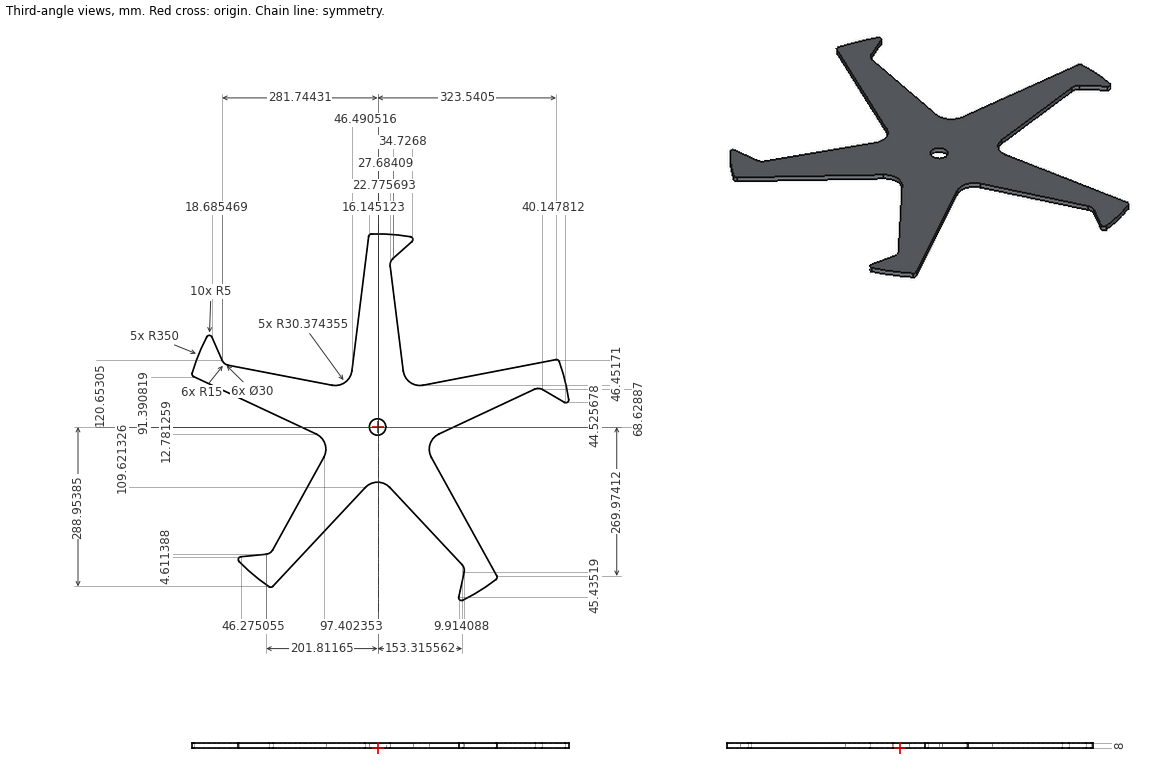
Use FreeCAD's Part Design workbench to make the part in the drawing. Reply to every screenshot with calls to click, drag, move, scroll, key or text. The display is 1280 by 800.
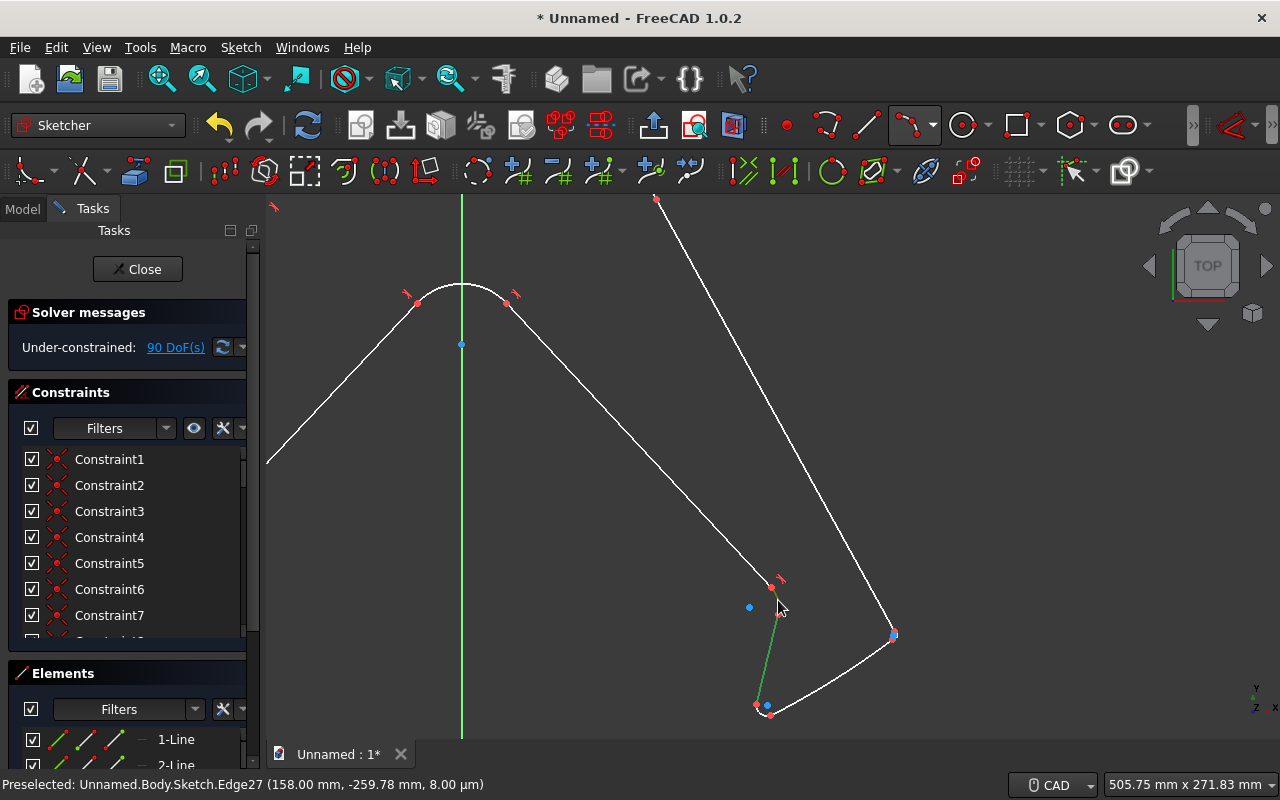
key(t)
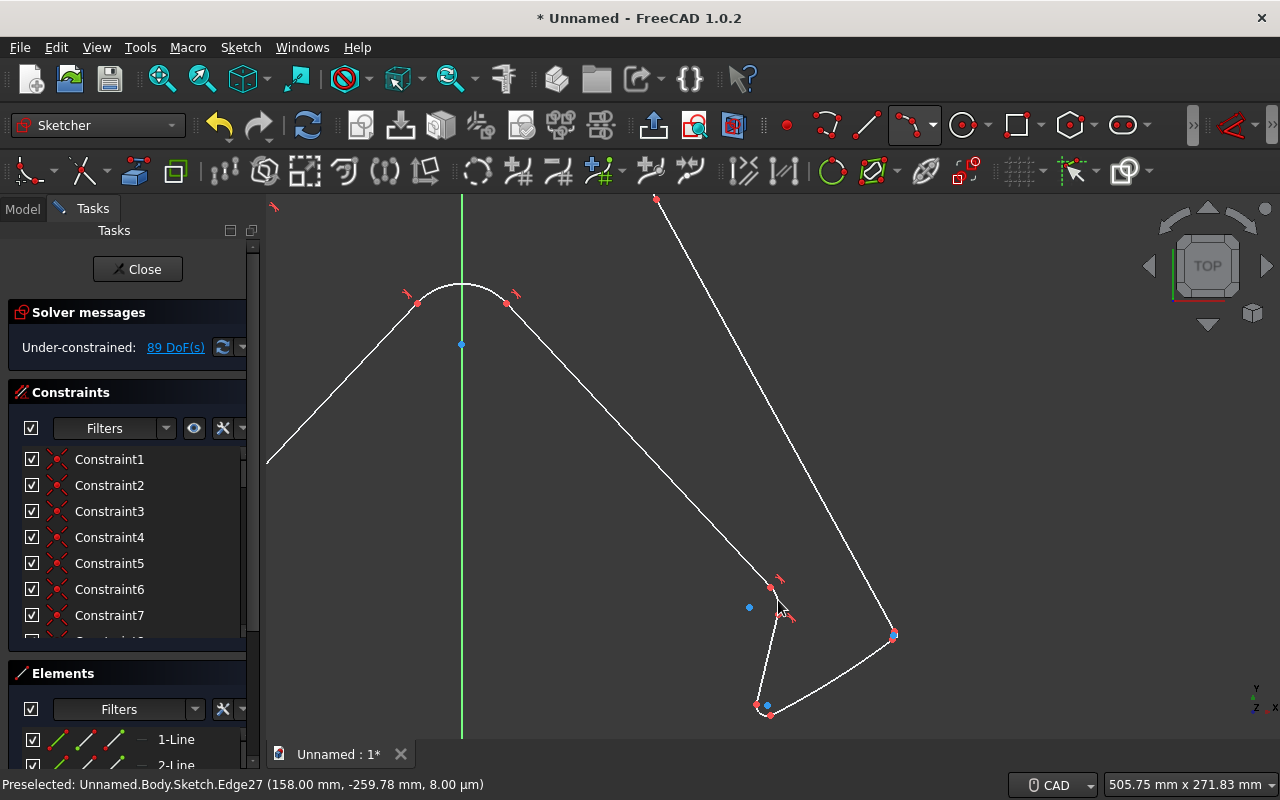
click(772, 641)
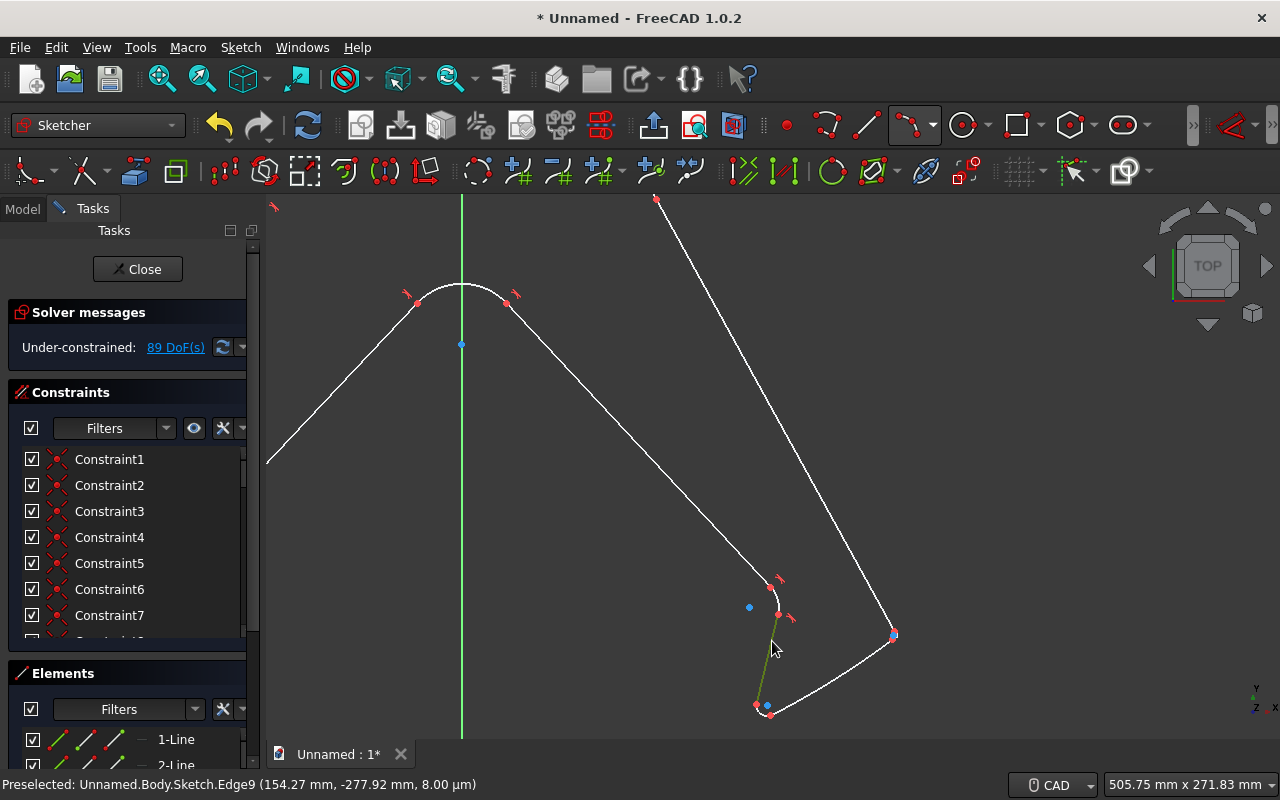
scroll(780, 603, down, 7)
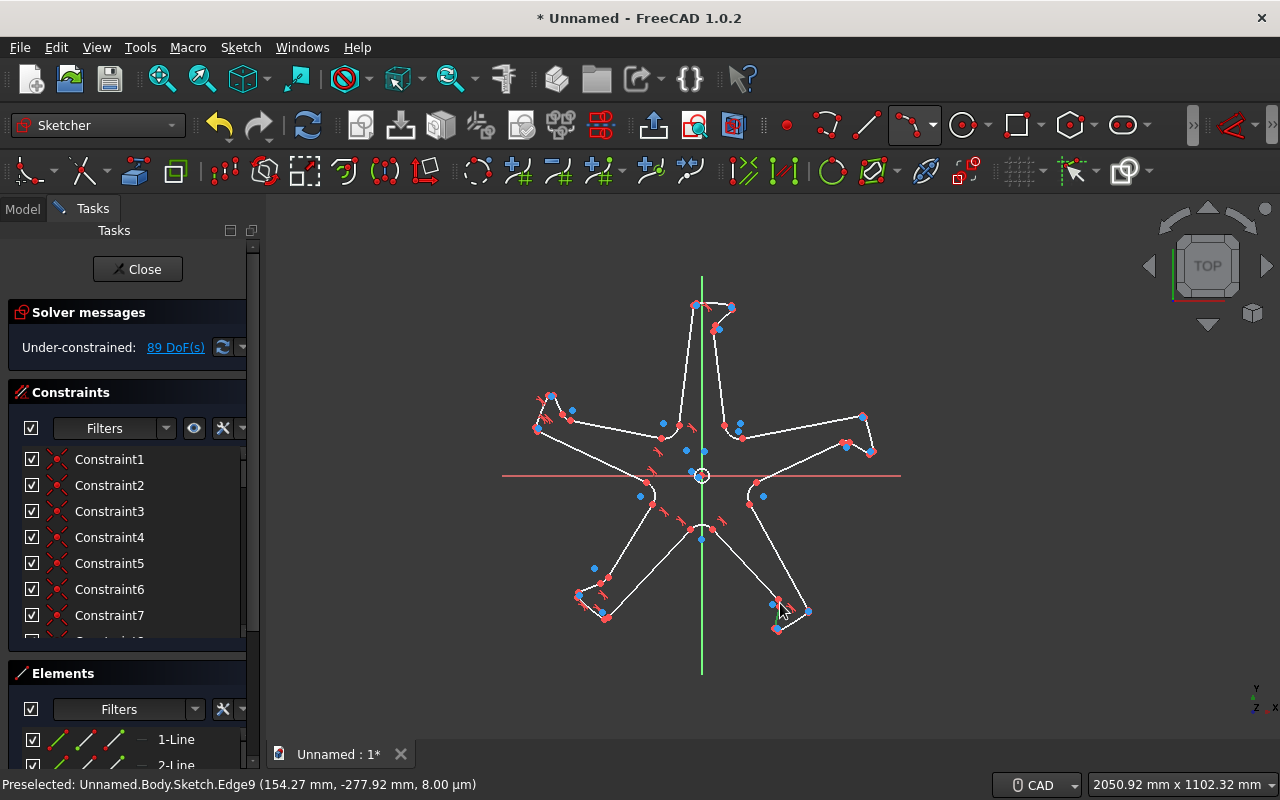
scroll(776, 631, up, 9)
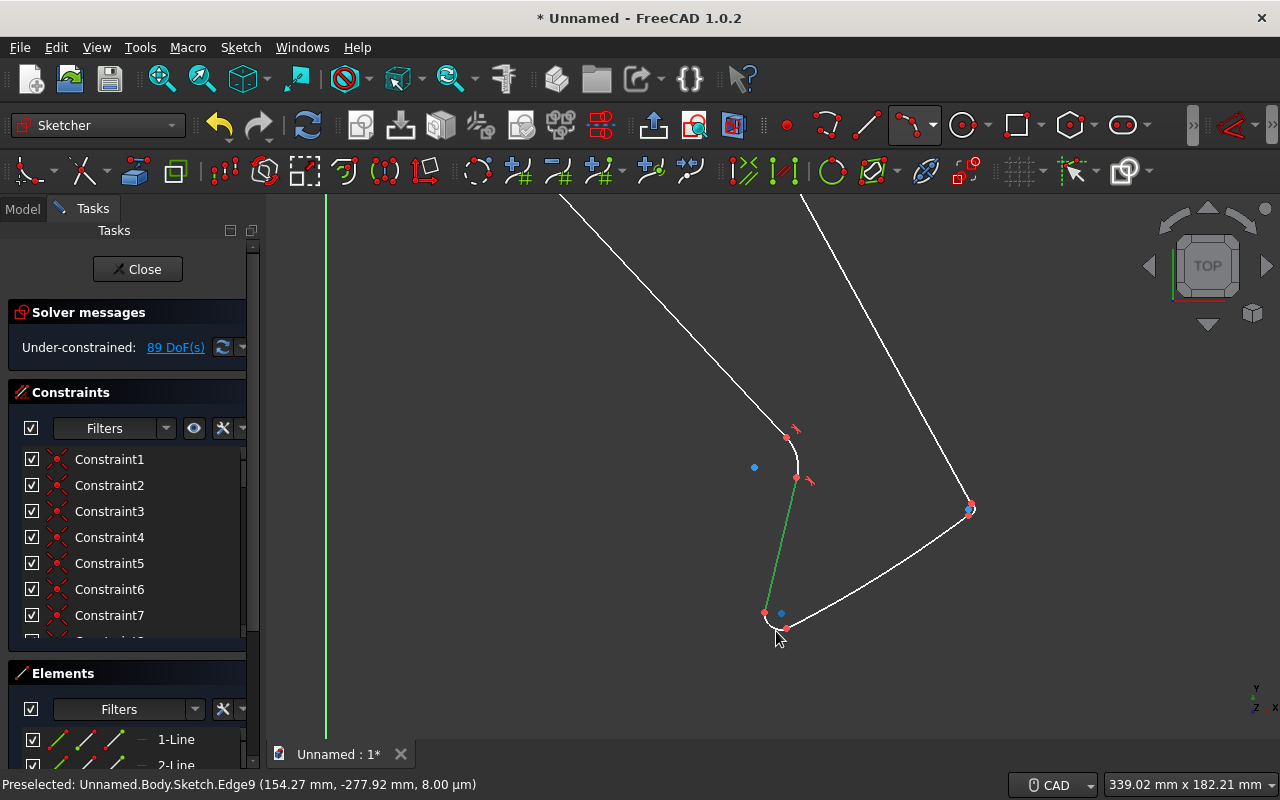
click(771, 627)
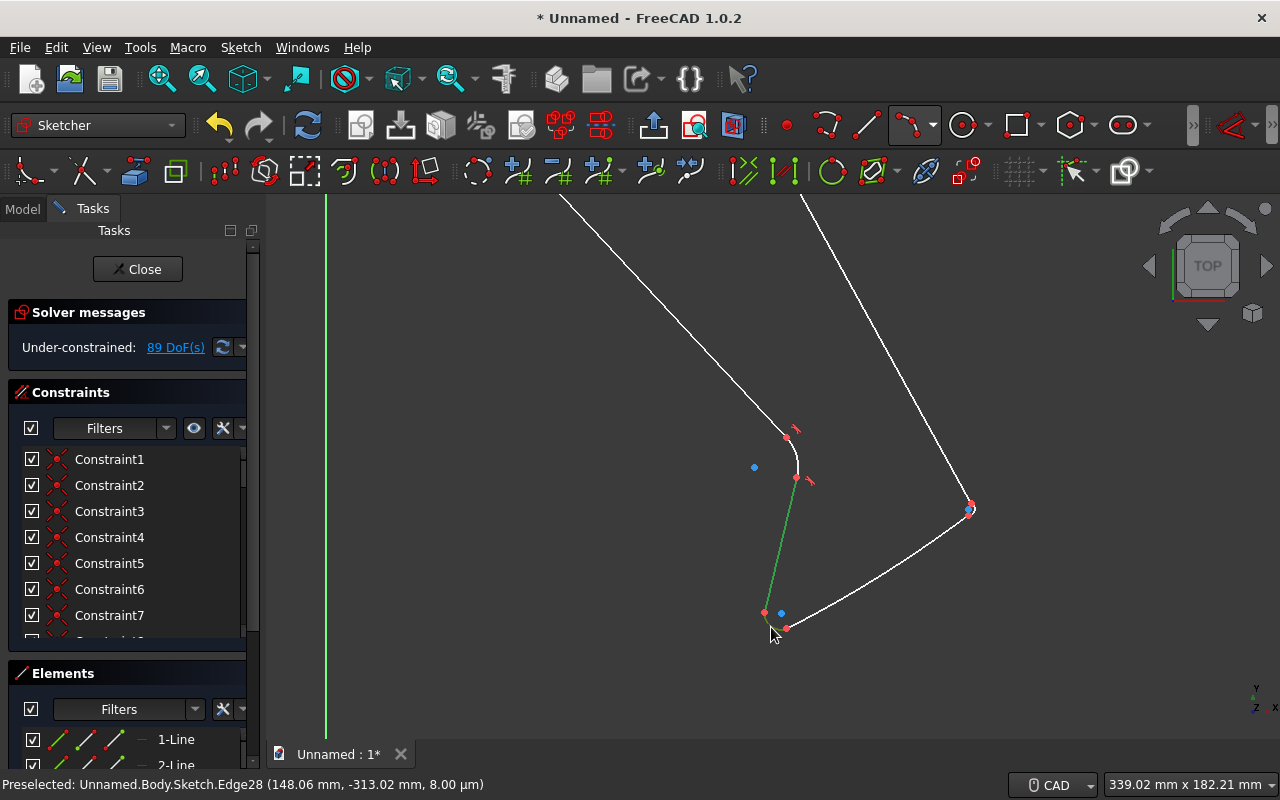
key(t)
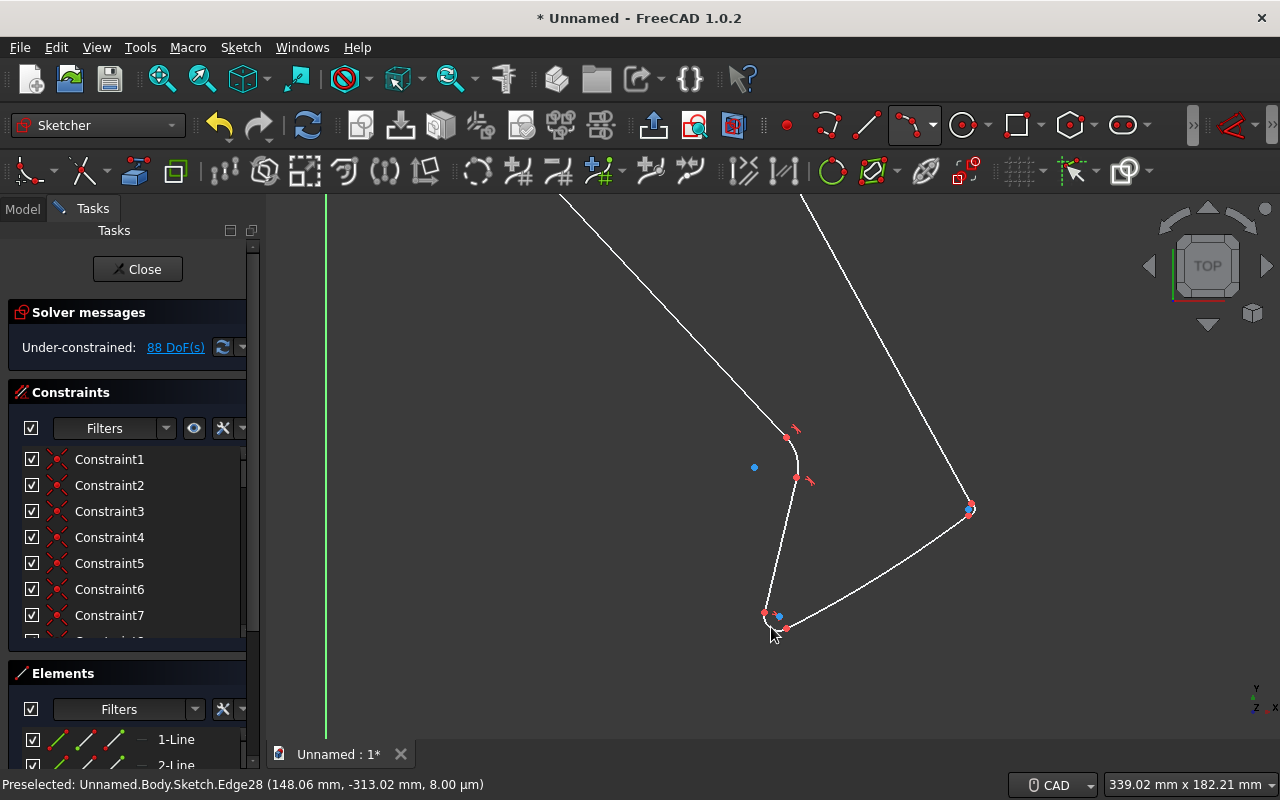
scroll(776, 631, down, 9)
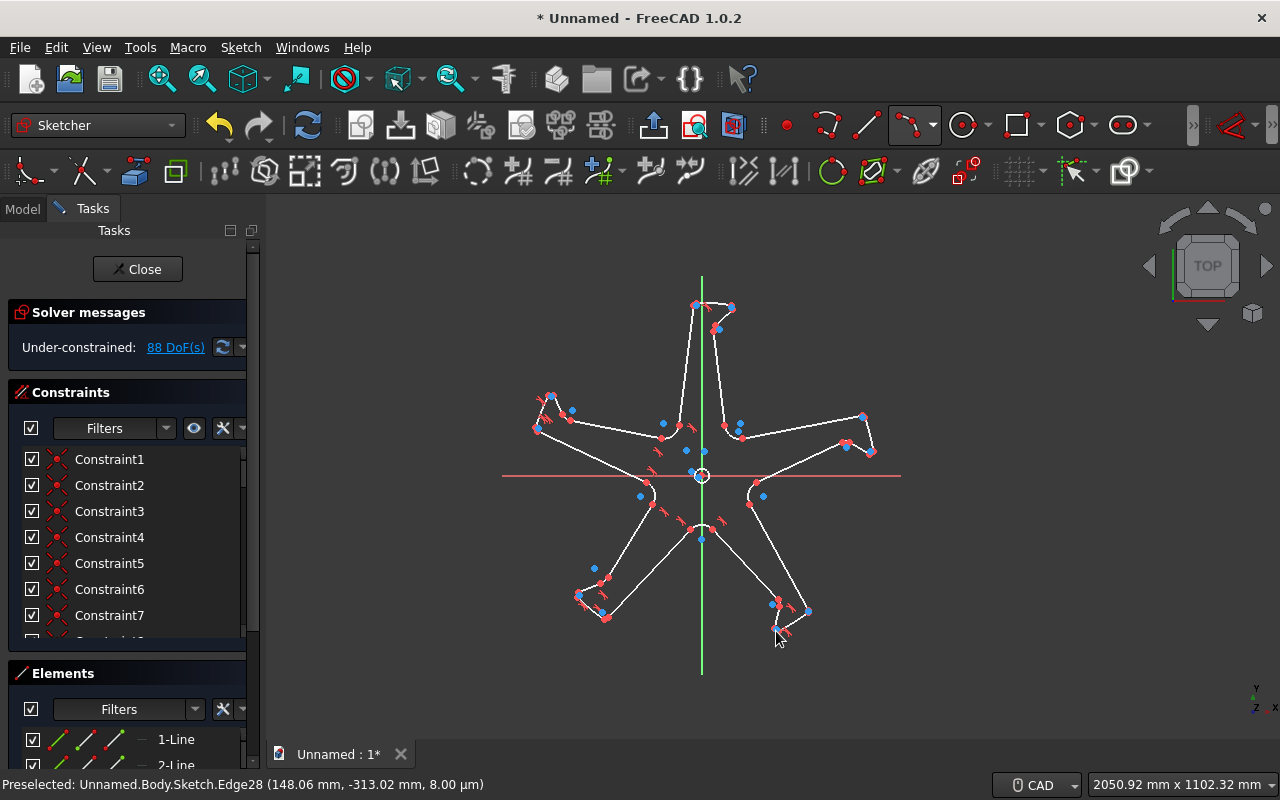
click(791, 579)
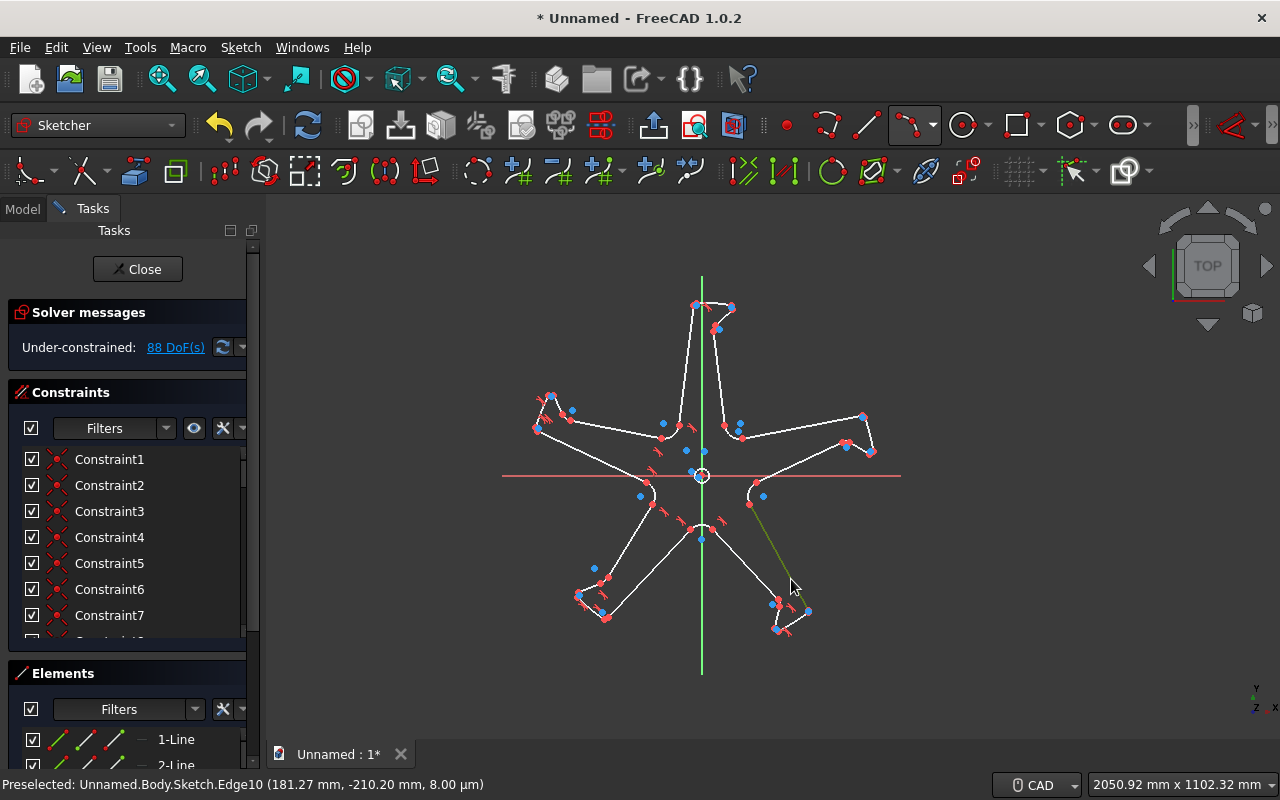
scroll(809, 612, up, 14)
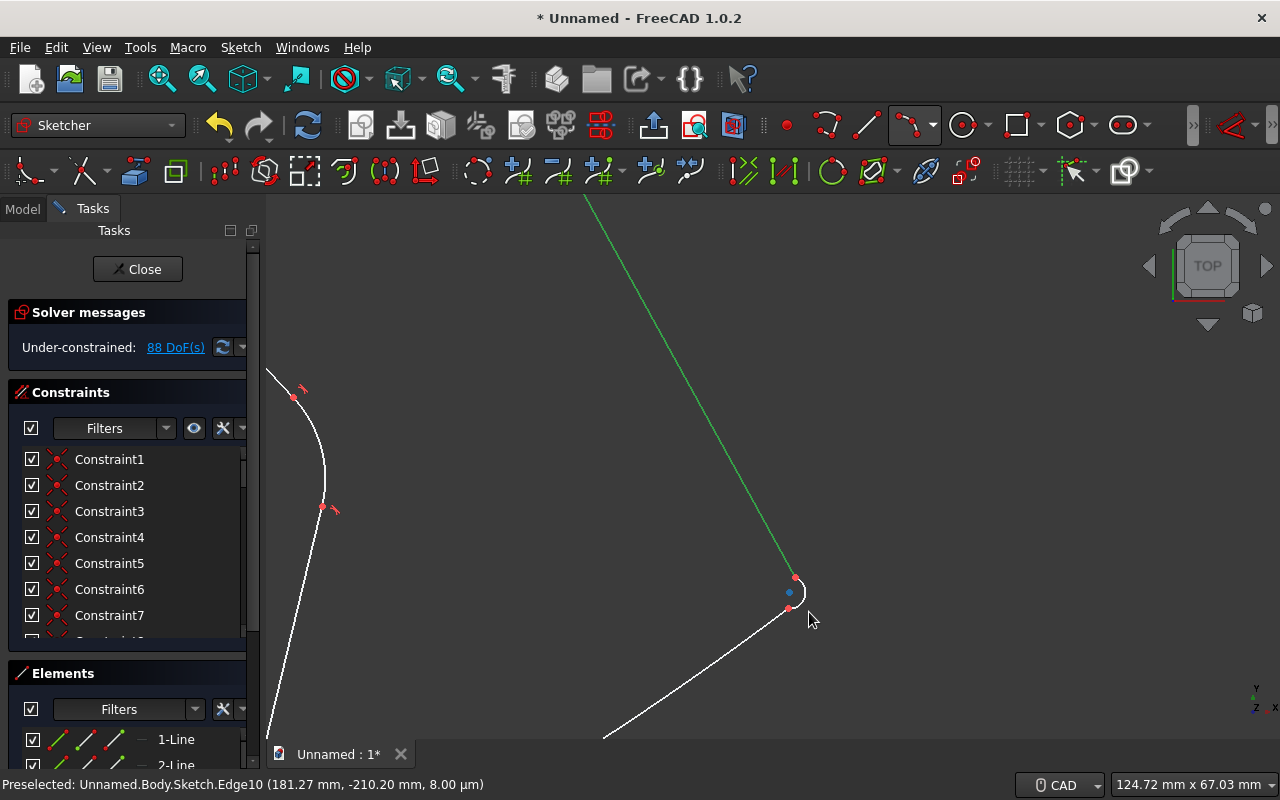
click(805, 596)